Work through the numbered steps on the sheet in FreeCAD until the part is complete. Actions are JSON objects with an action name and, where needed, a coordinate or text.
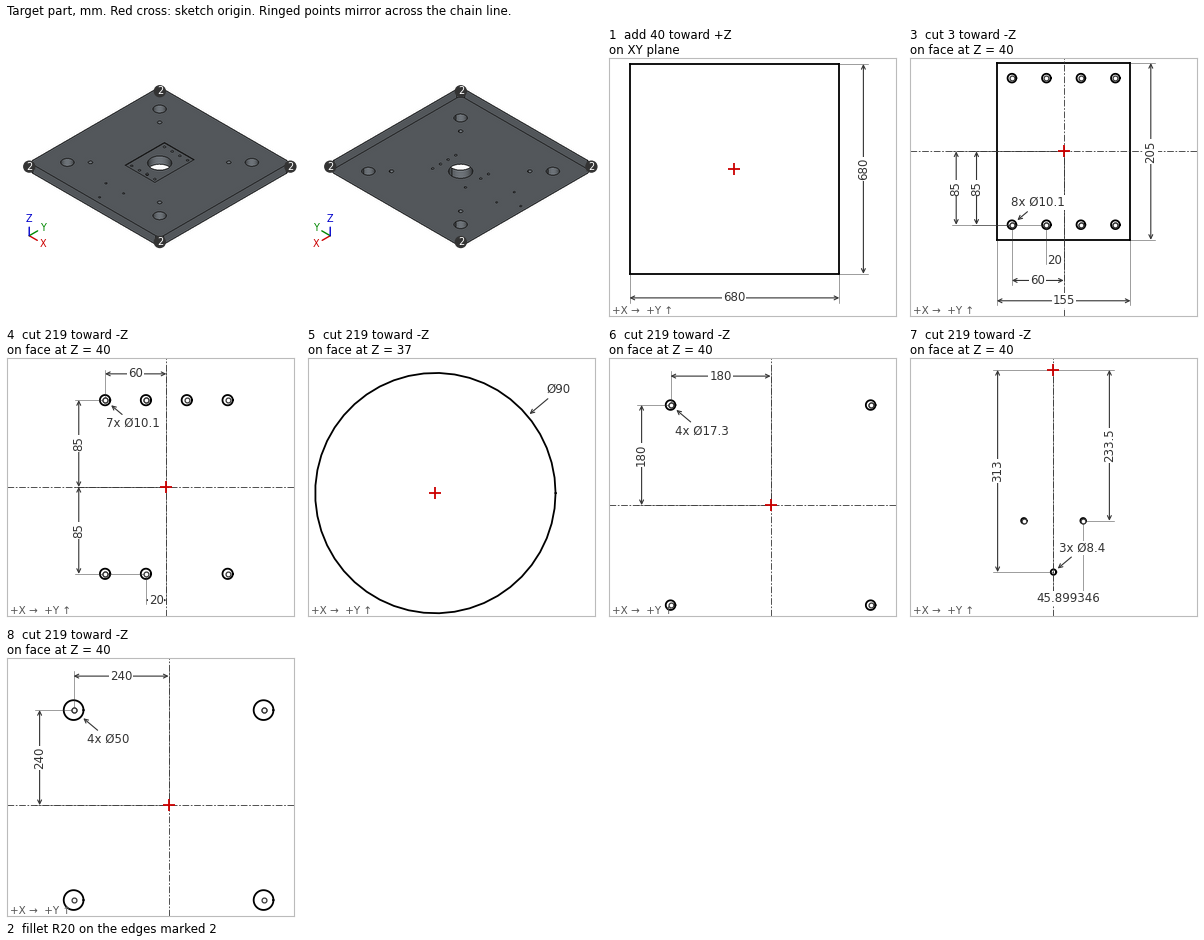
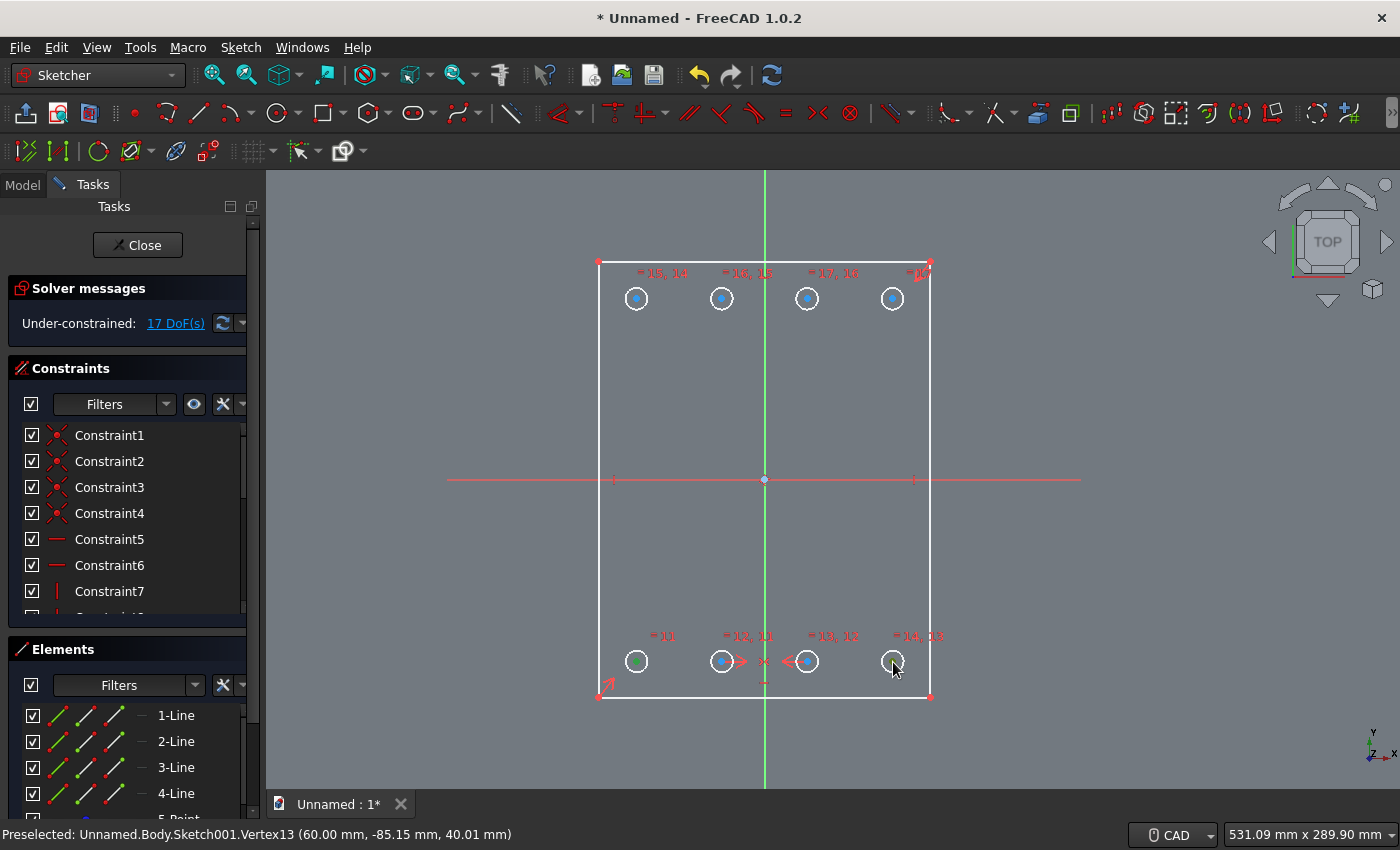
{"action": "left_click", "coordinate": [765, 600]}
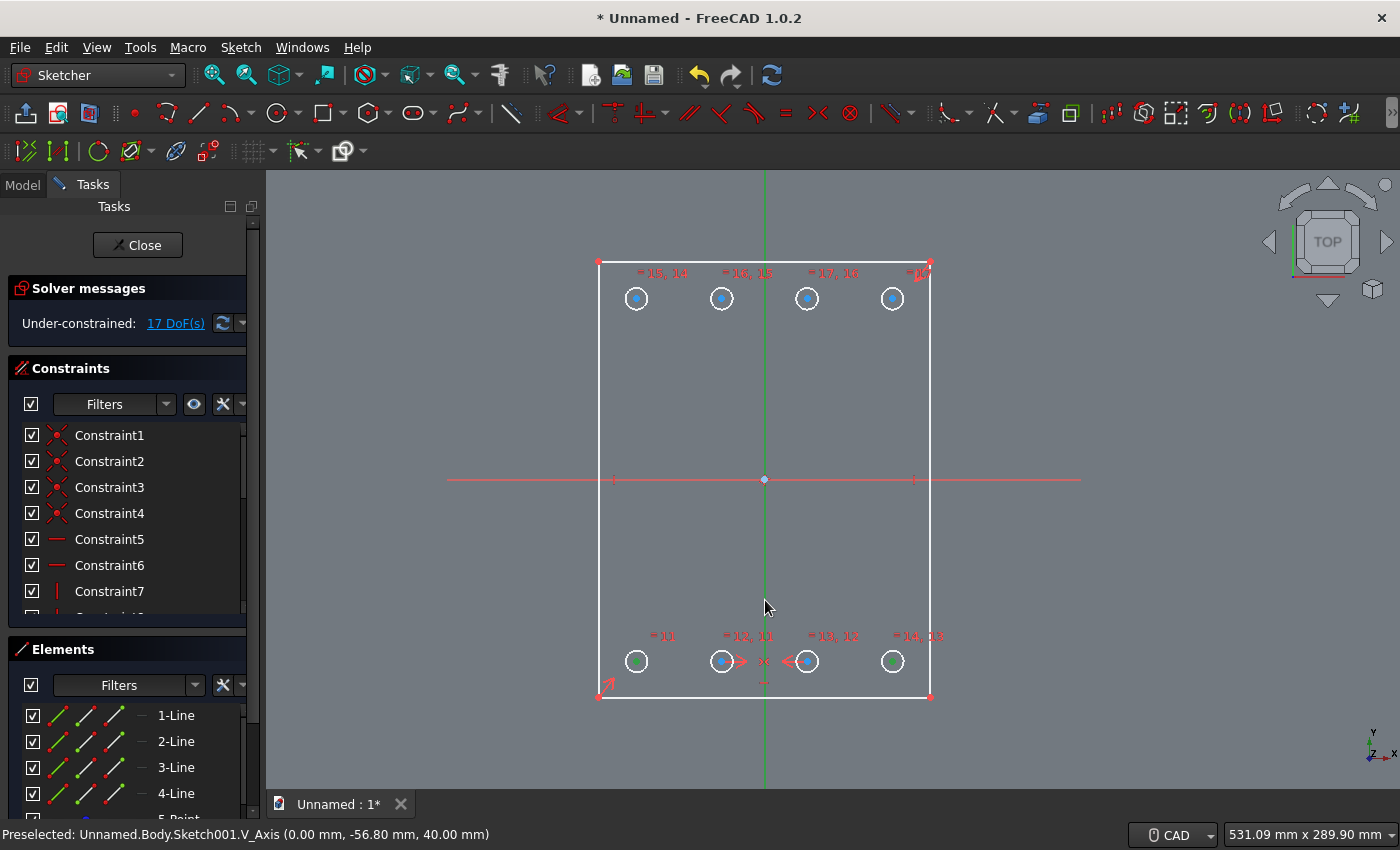
{"action": "left_click", "coordinate": [818, 114]}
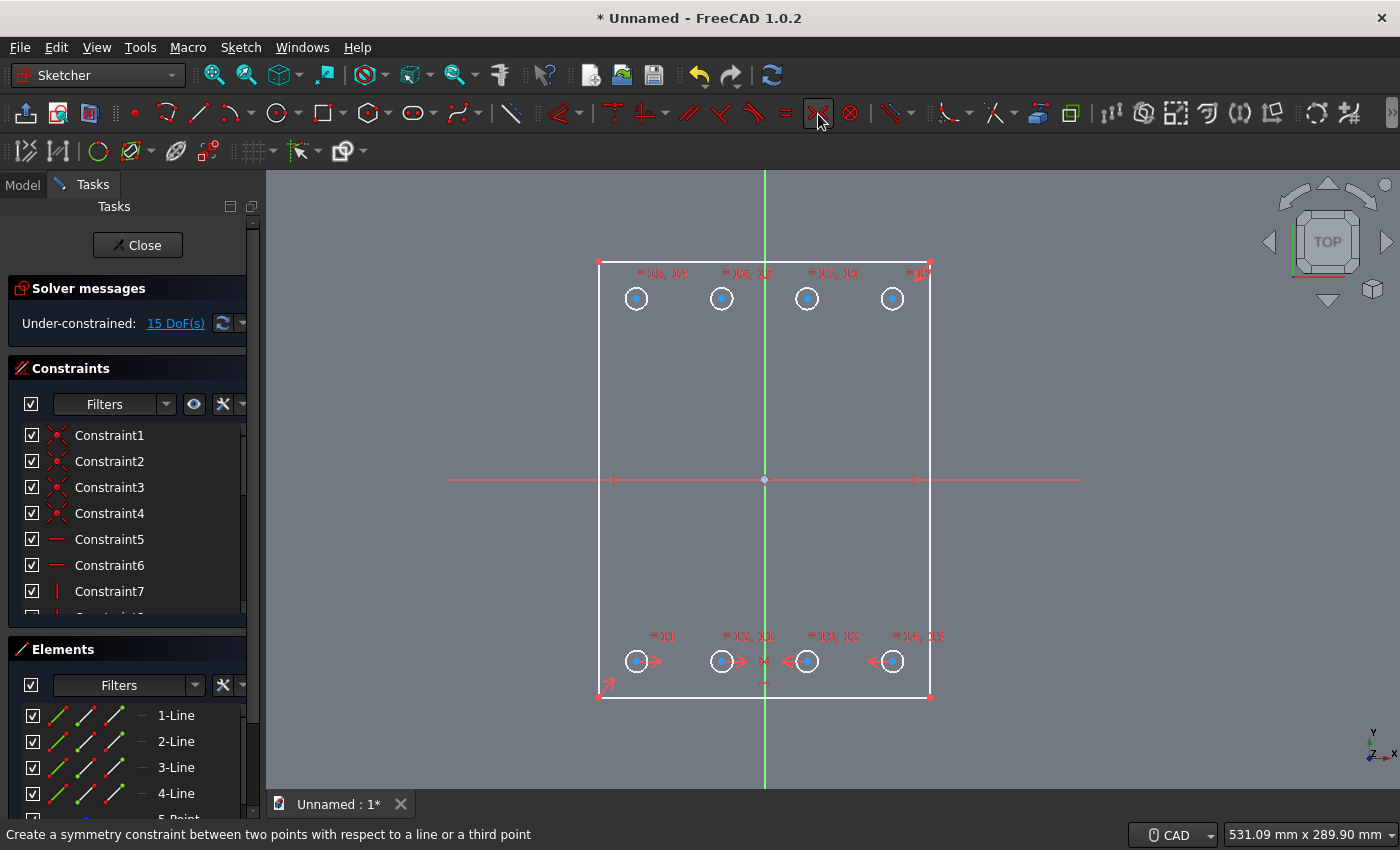
{"action": "left_click", "coordinate": [637, 662]}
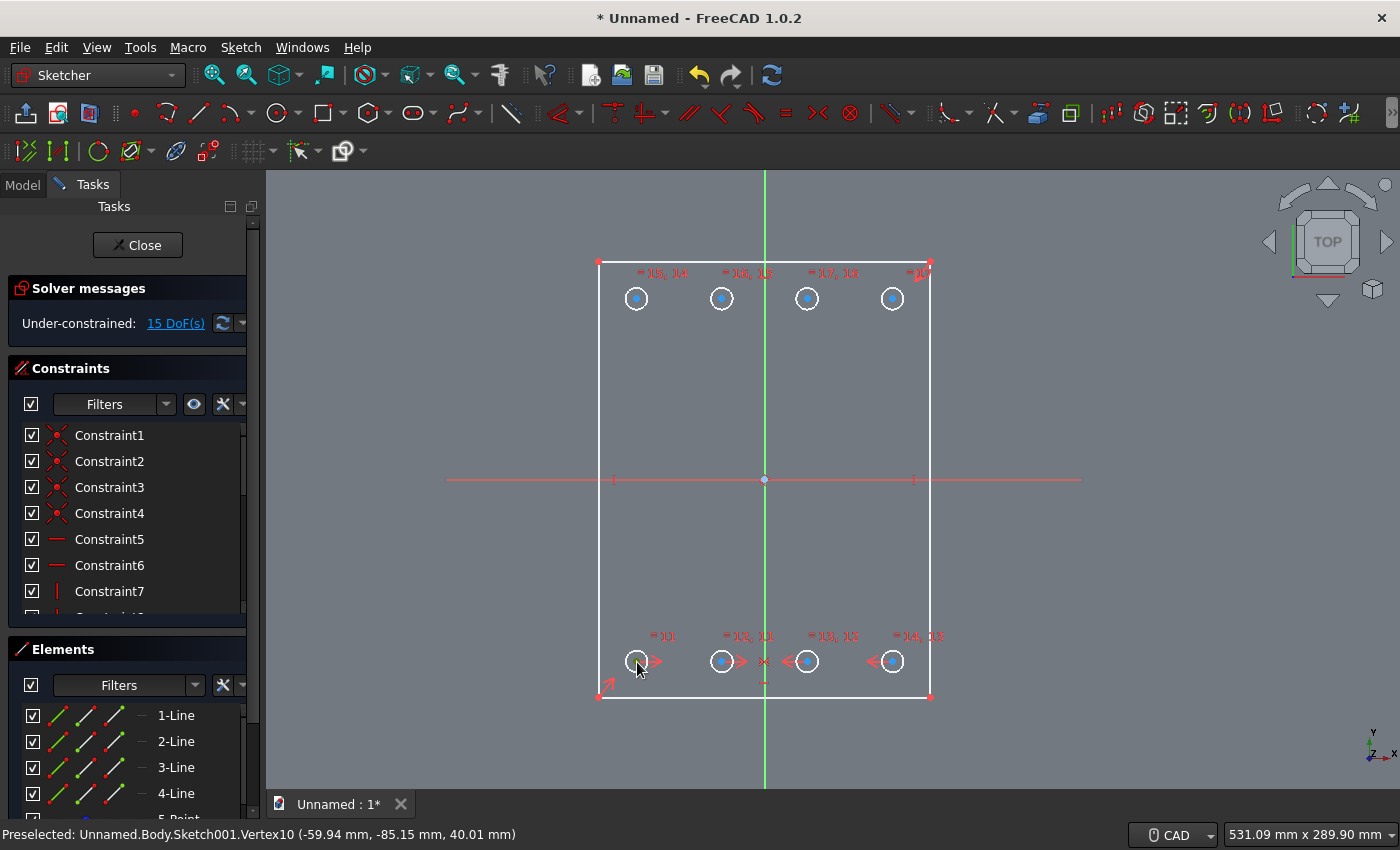
{"action": "left_click", "coordinate": [636, 299]}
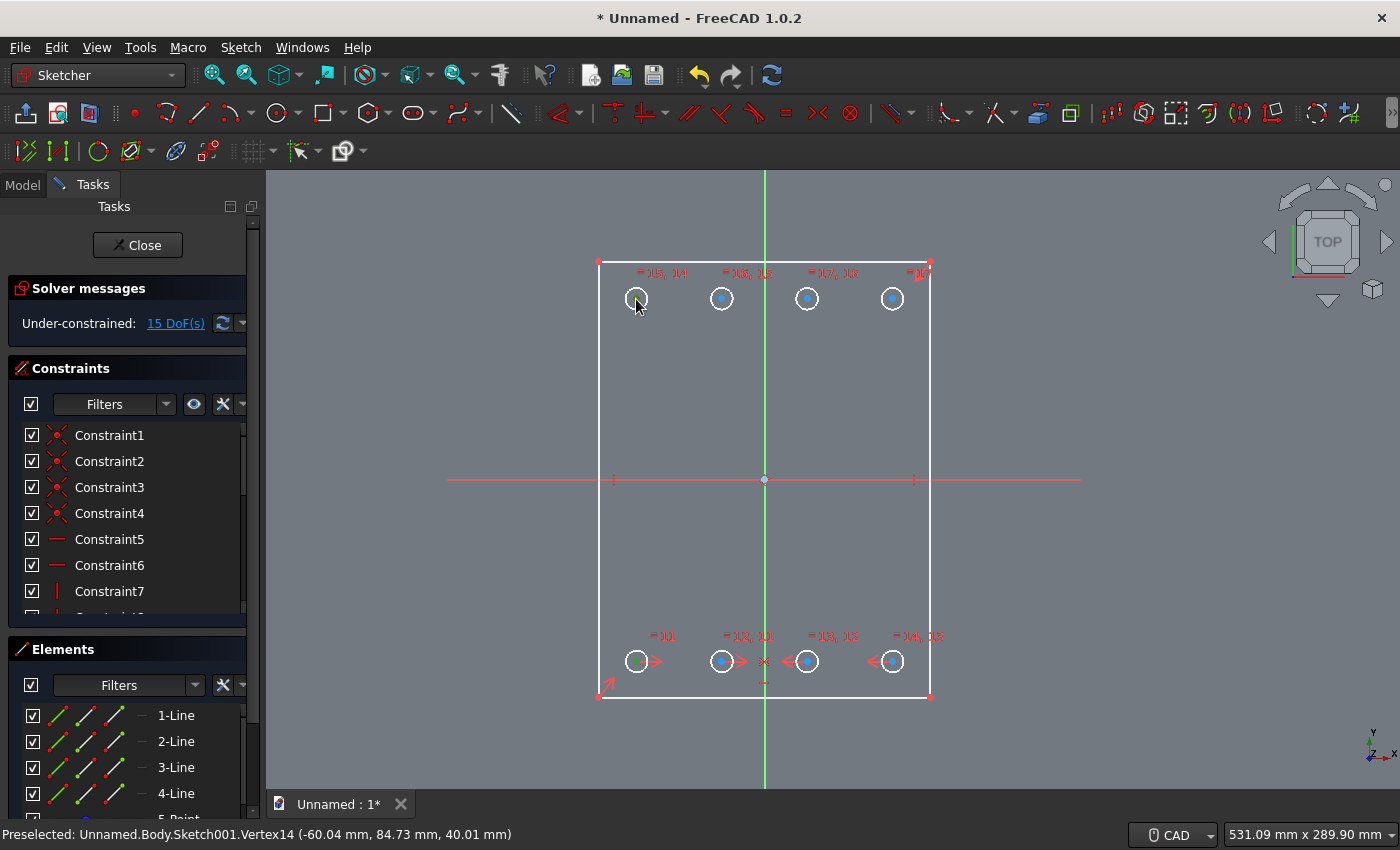
{"action": "left_click", "coordinate": [496, 480]}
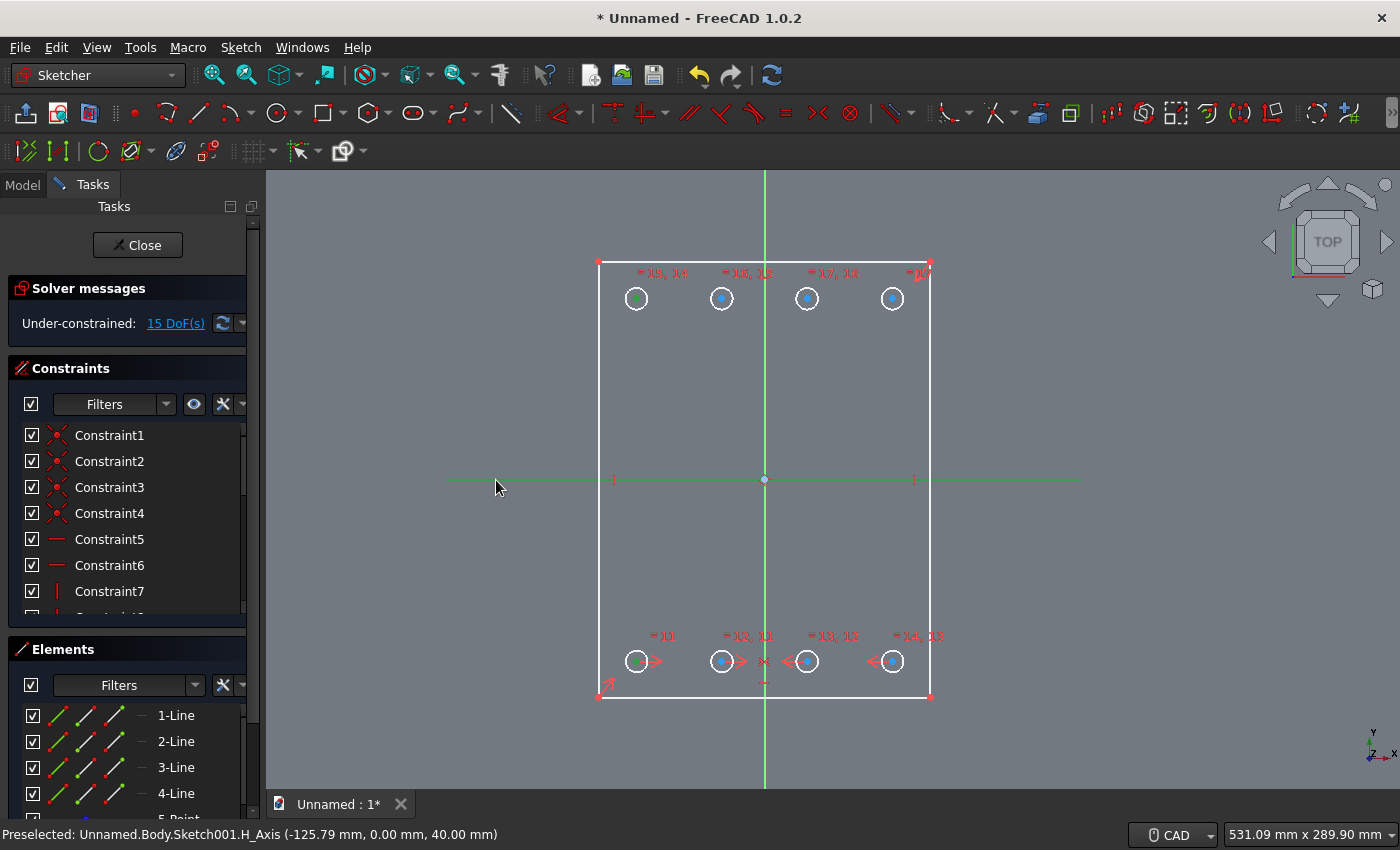
{"action": "left_click", "coordinate": [818, 114]}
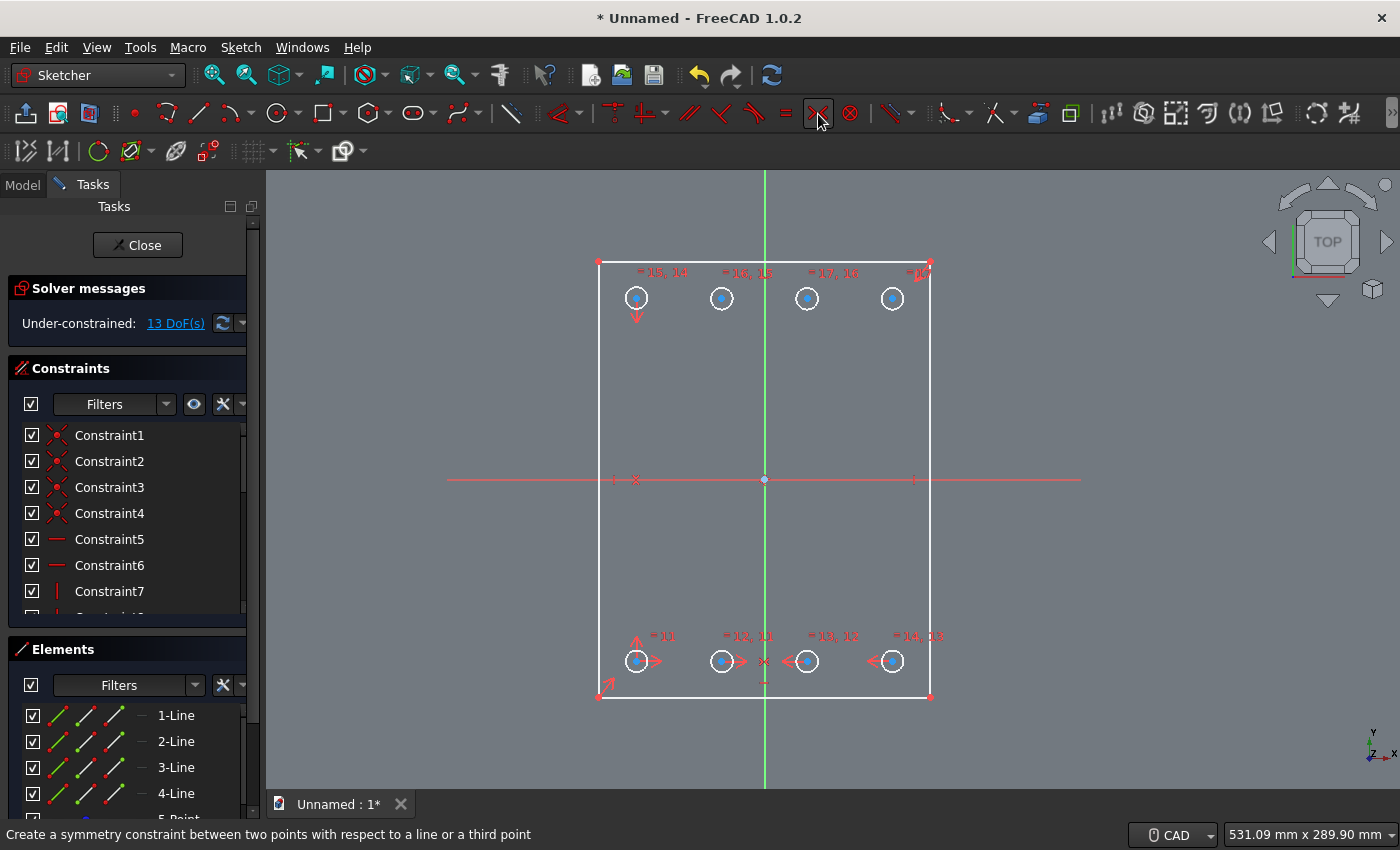
{"action": "left_click", "coordinate": [722, 662]}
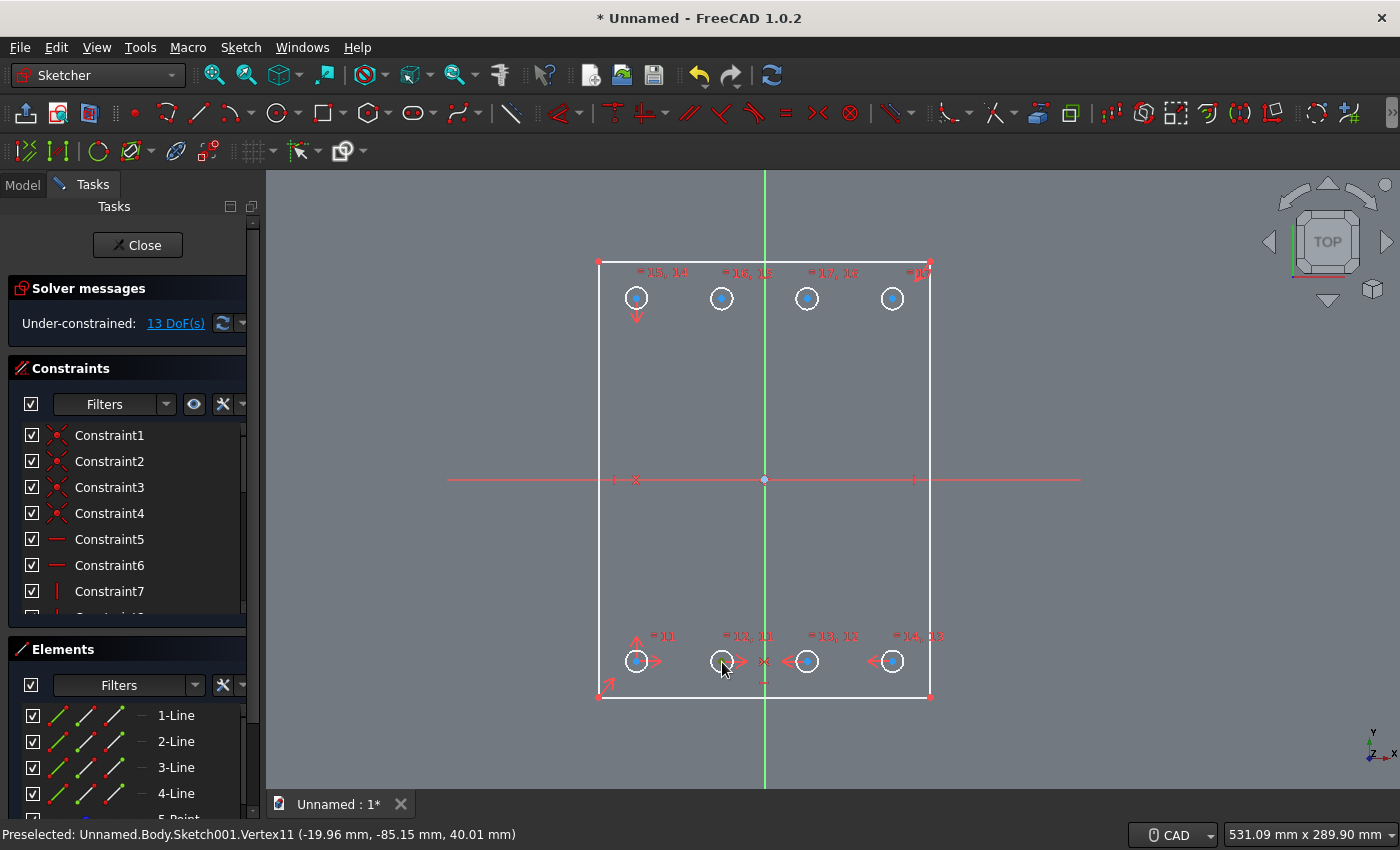
{"action": "left_click", "coordinate": [722, 299]}